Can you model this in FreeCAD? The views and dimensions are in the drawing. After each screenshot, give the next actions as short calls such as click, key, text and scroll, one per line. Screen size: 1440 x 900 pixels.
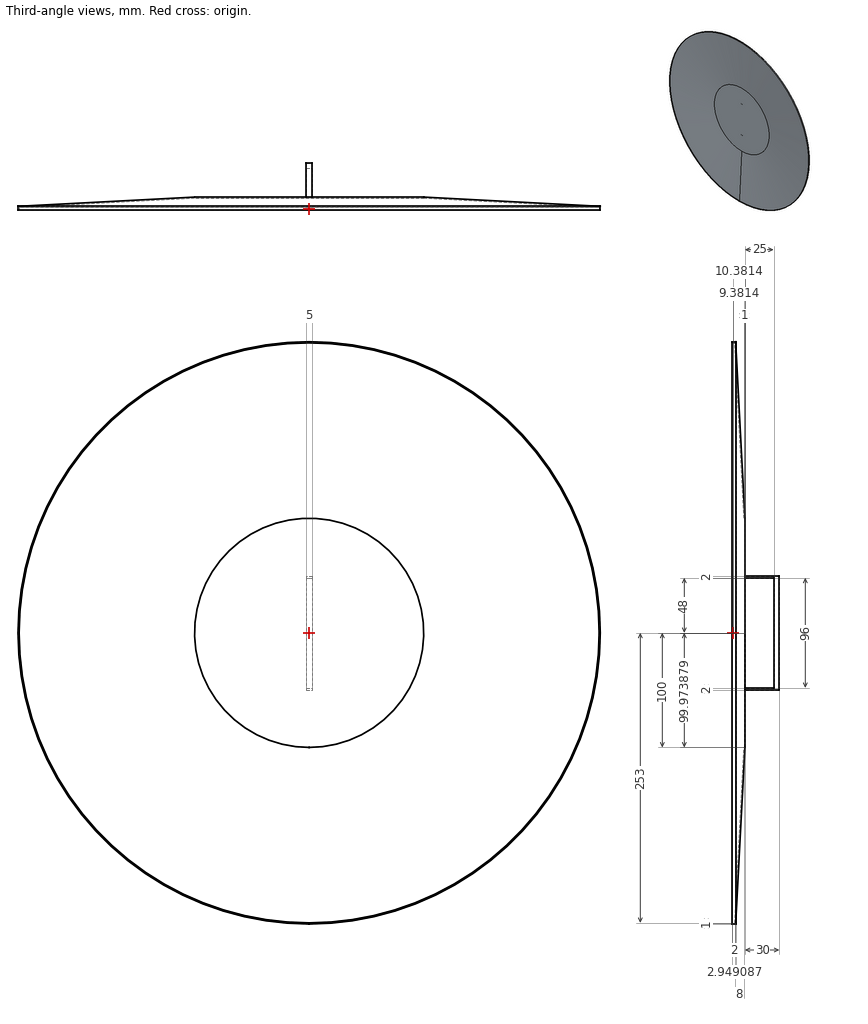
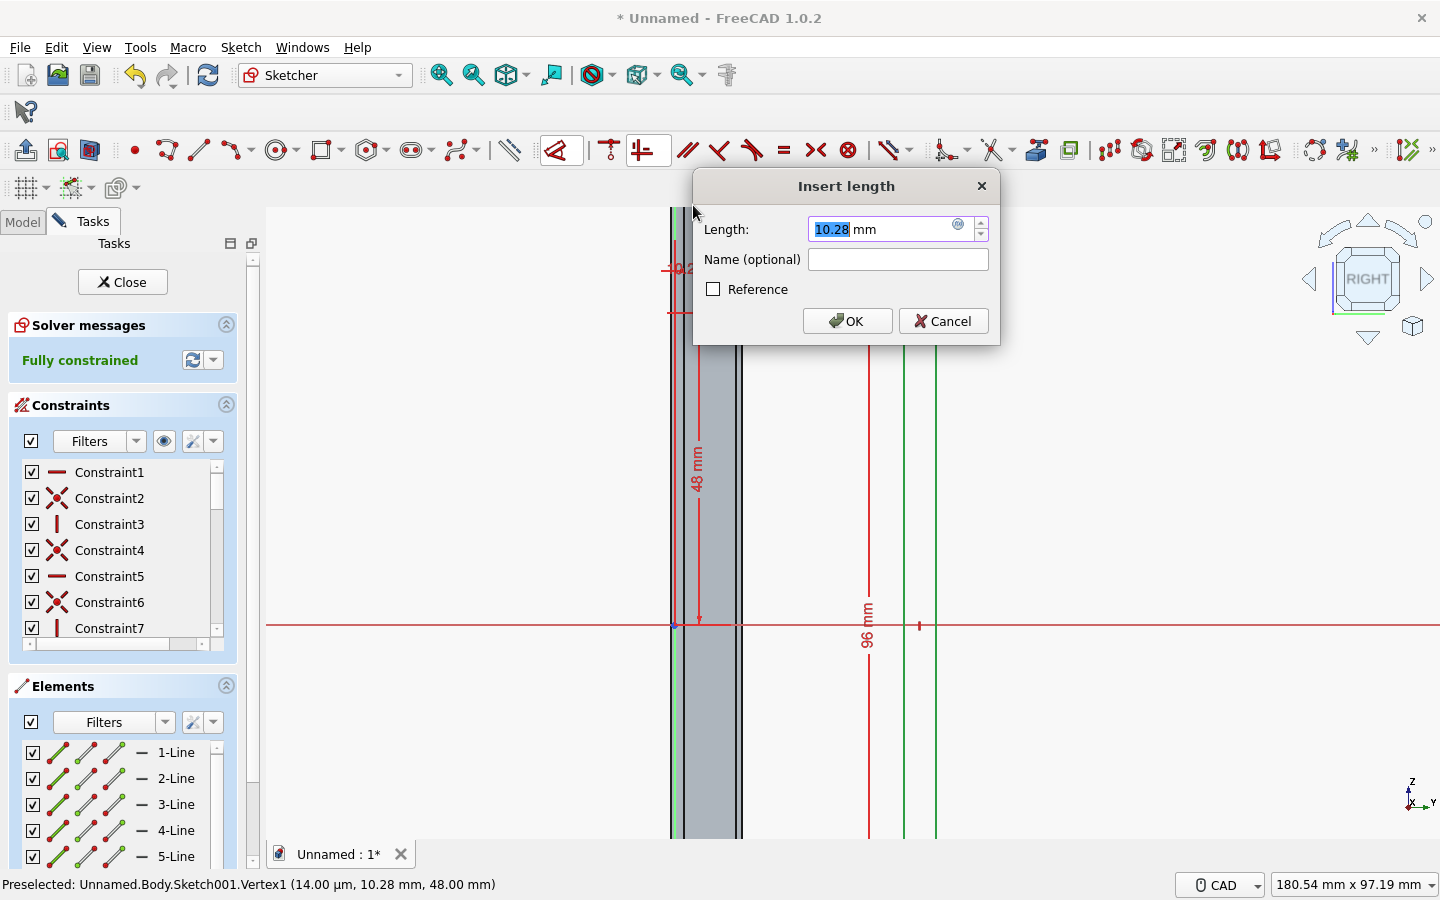
text(10.3814)
key(Return)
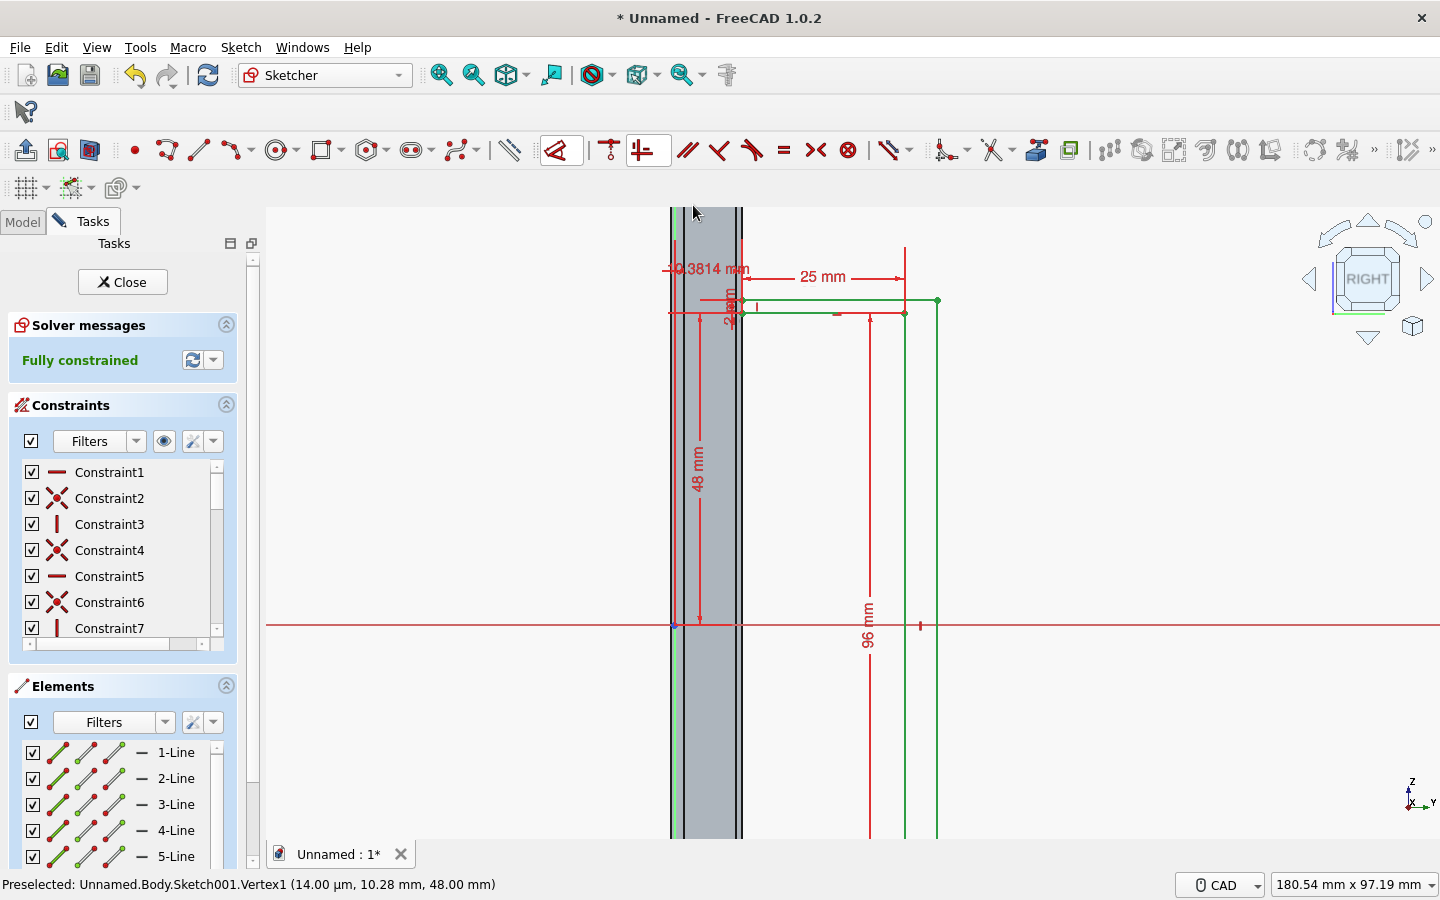
click(123, 282)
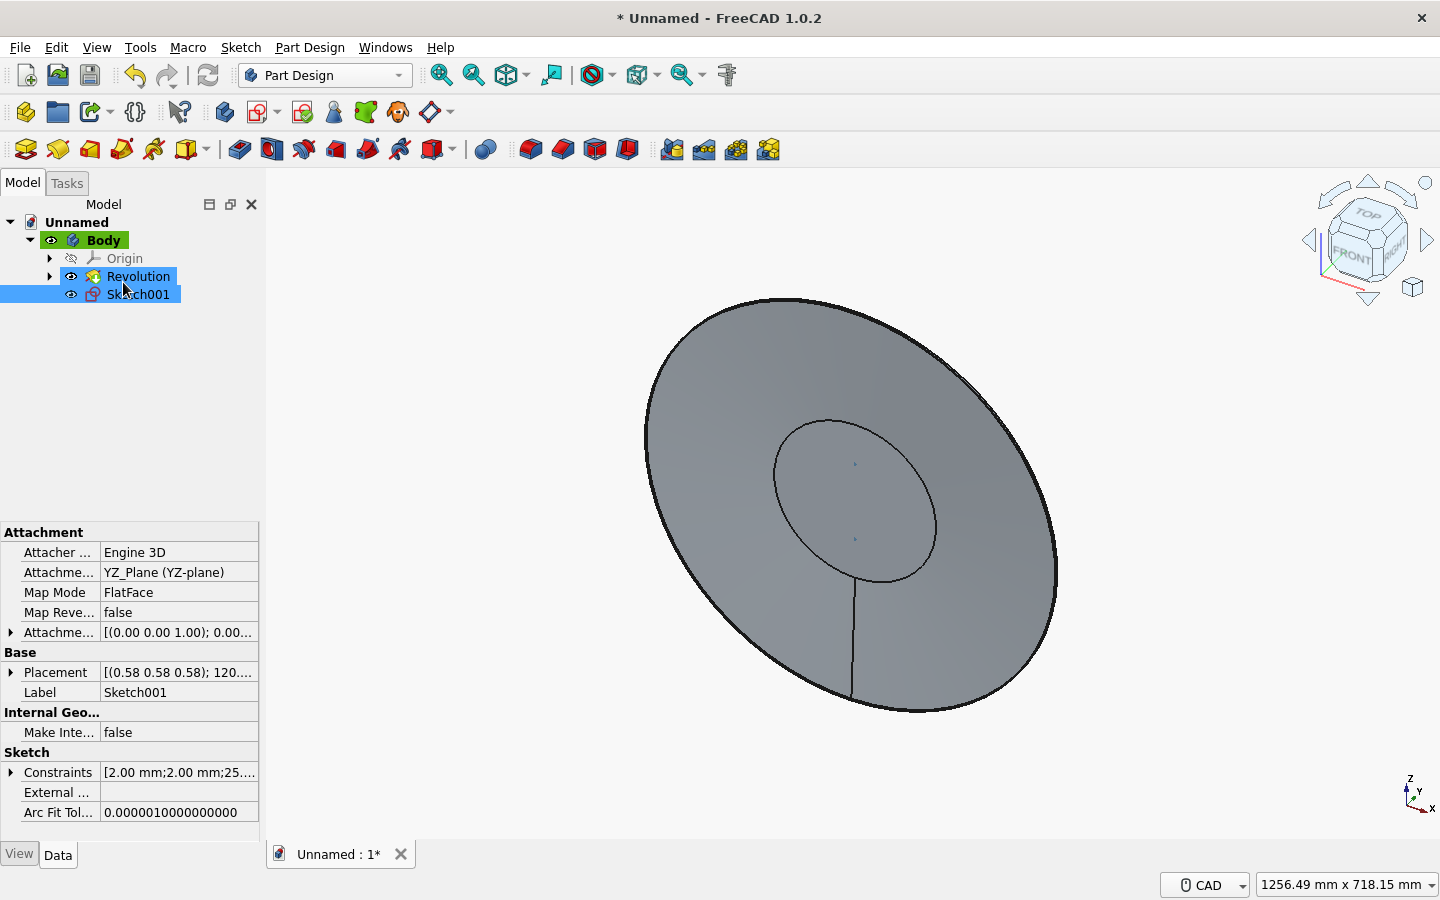
click(26, 150)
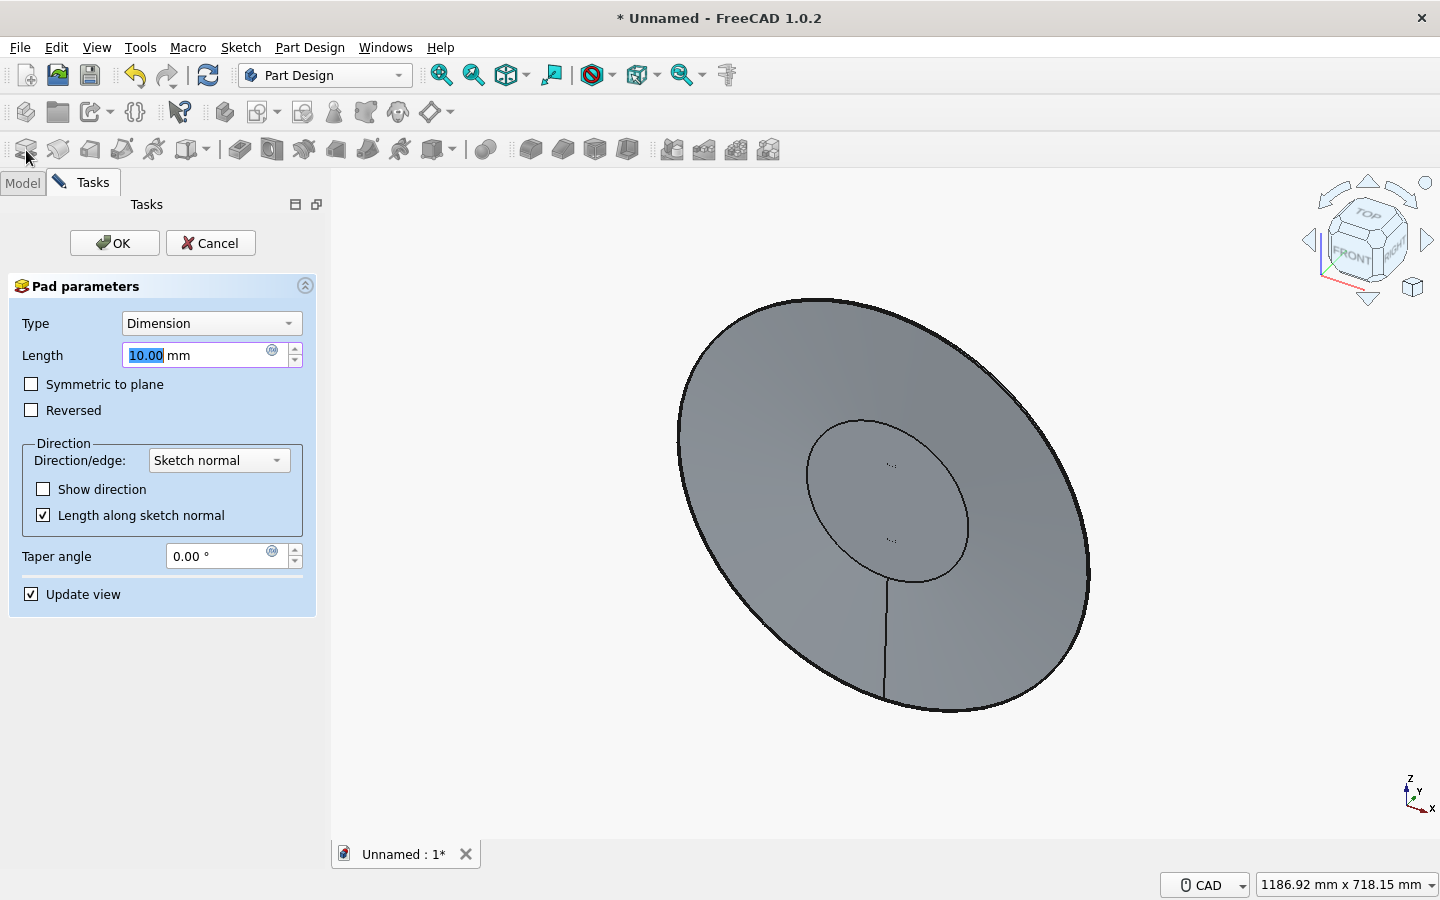
text(5)
key(Tab)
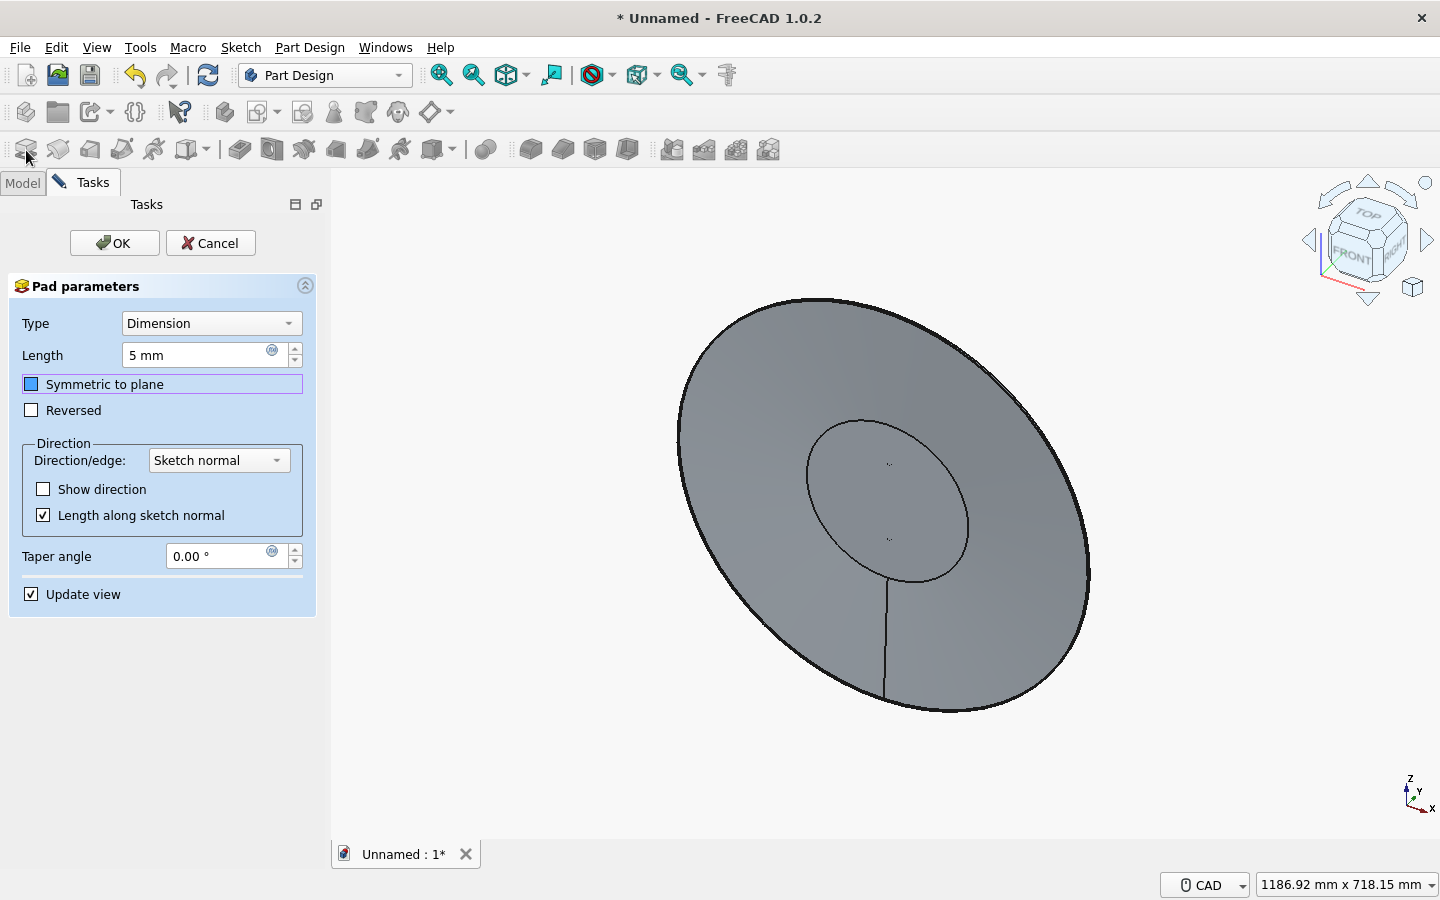
click(30, 384)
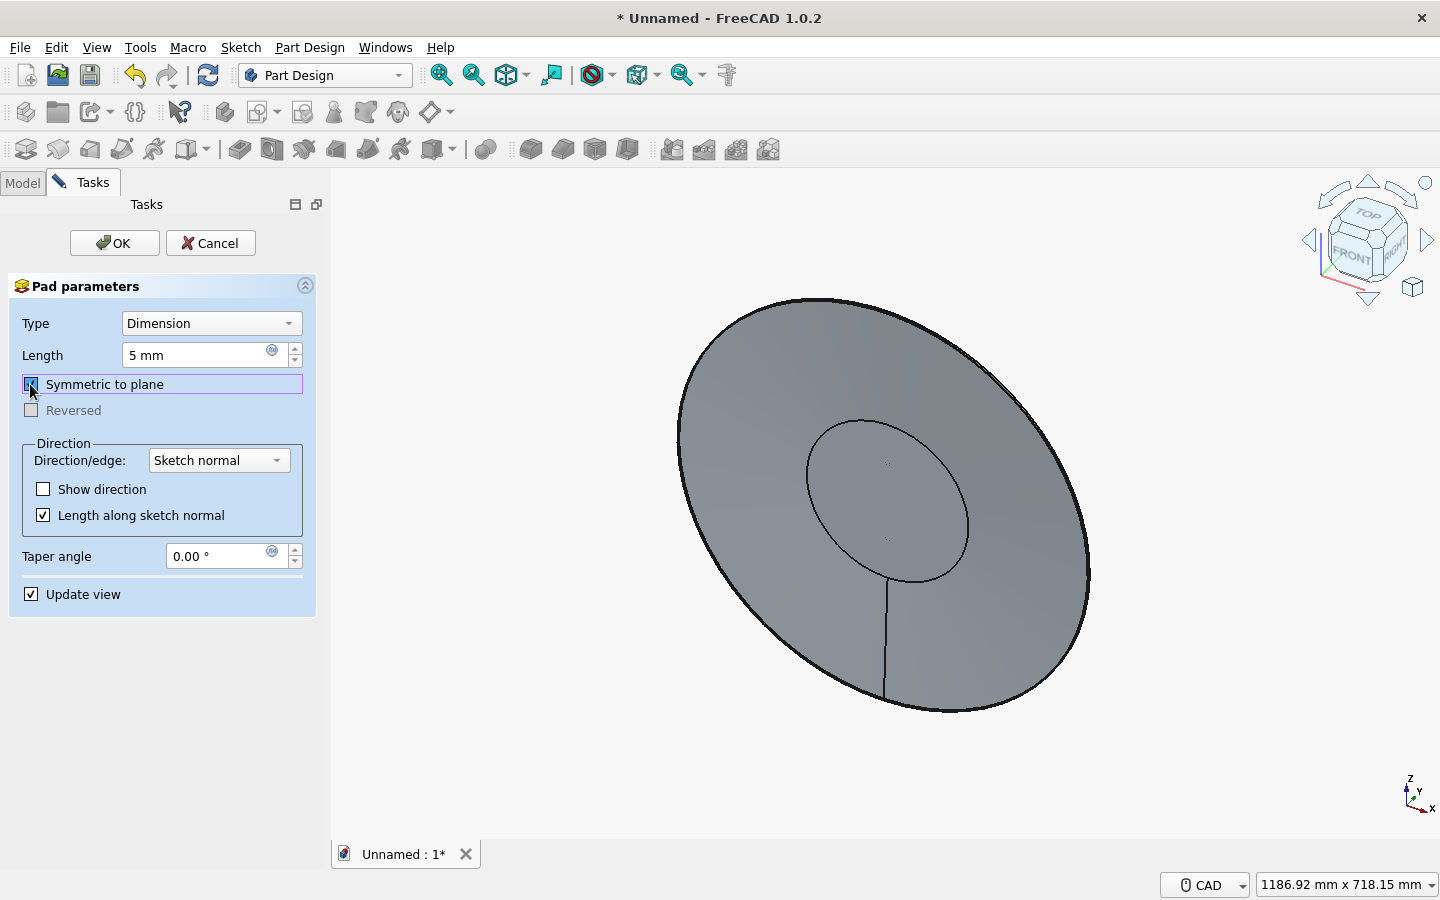
click(115, 243)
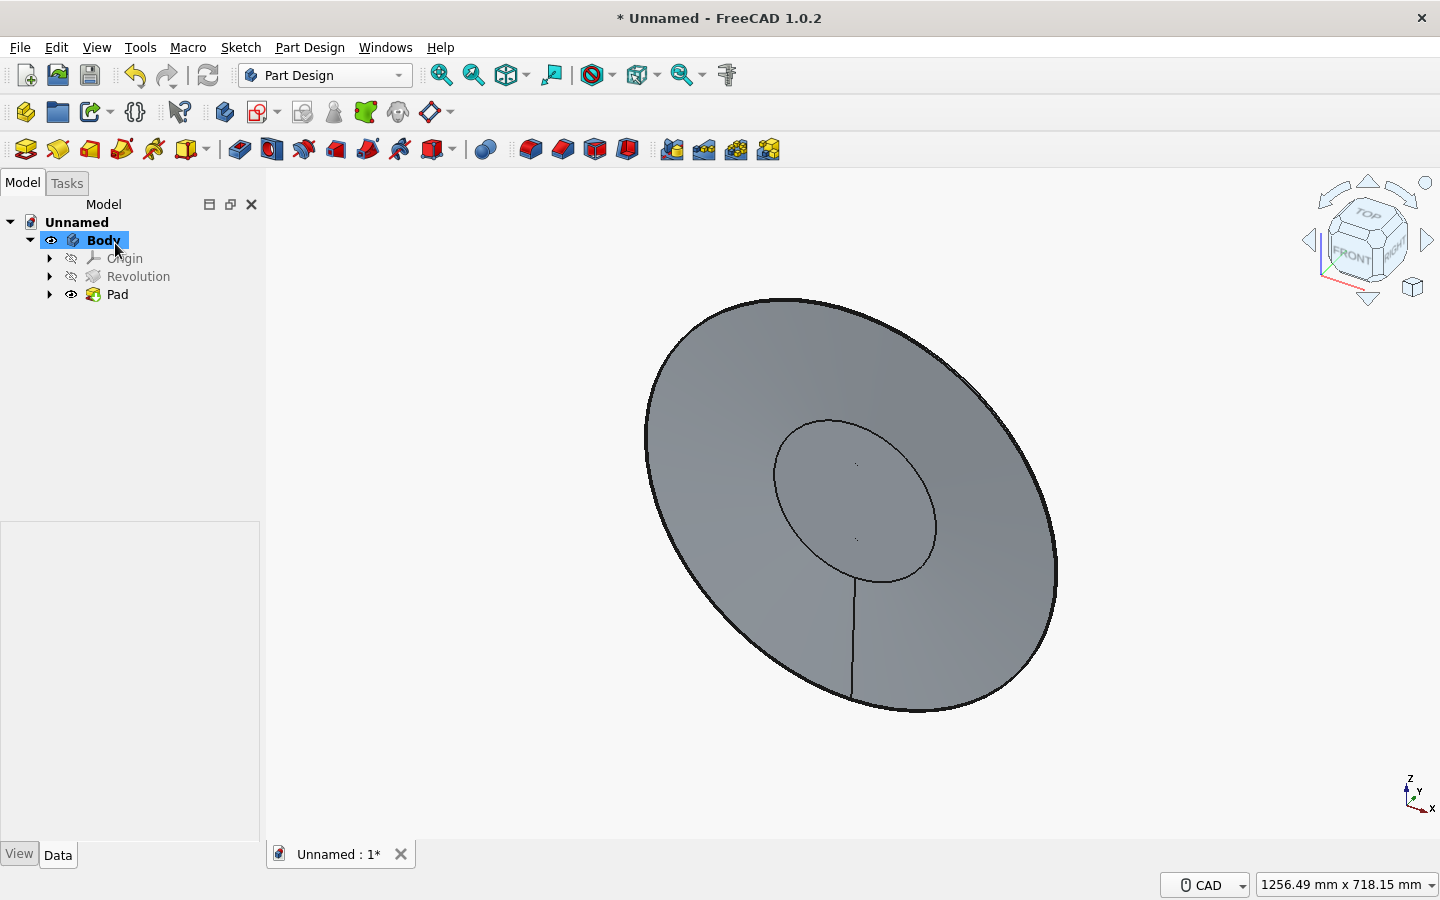
key(0)